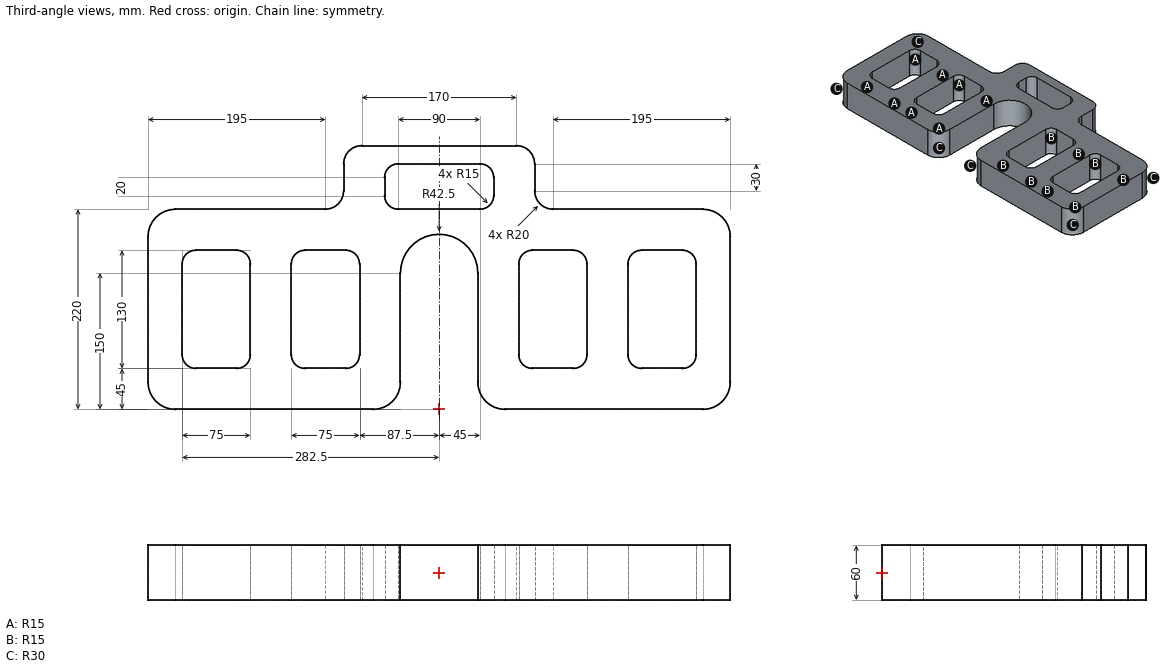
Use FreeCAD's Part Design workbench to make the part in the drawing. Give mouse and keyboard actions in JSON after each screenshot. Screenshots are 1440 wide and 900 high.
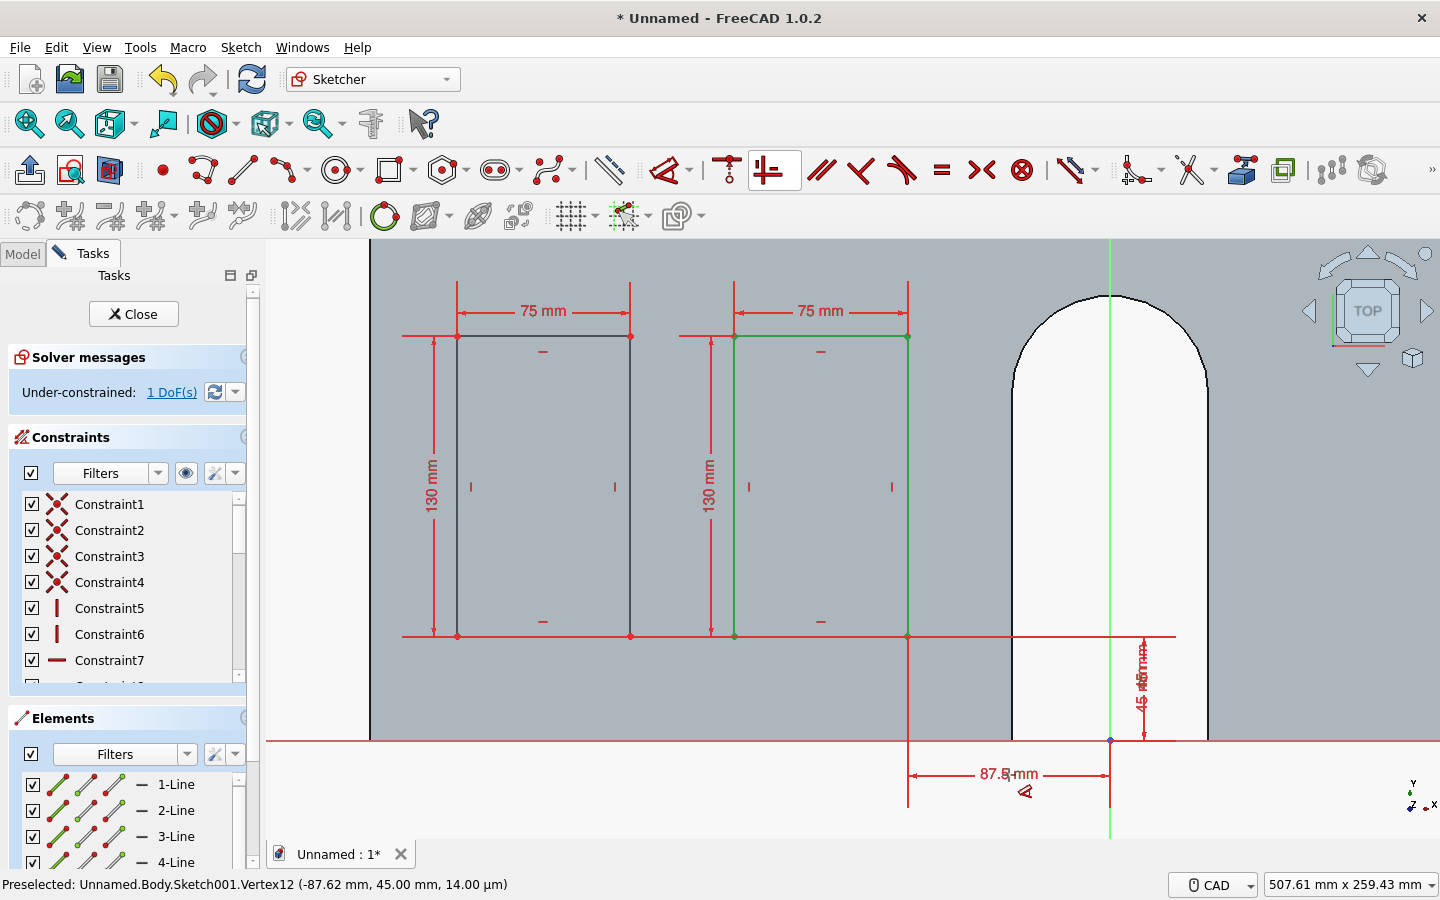
{"action": "left_click", "coordinate": [457, 336]}
{"action": "left_click", "coordinate": [784, 775]}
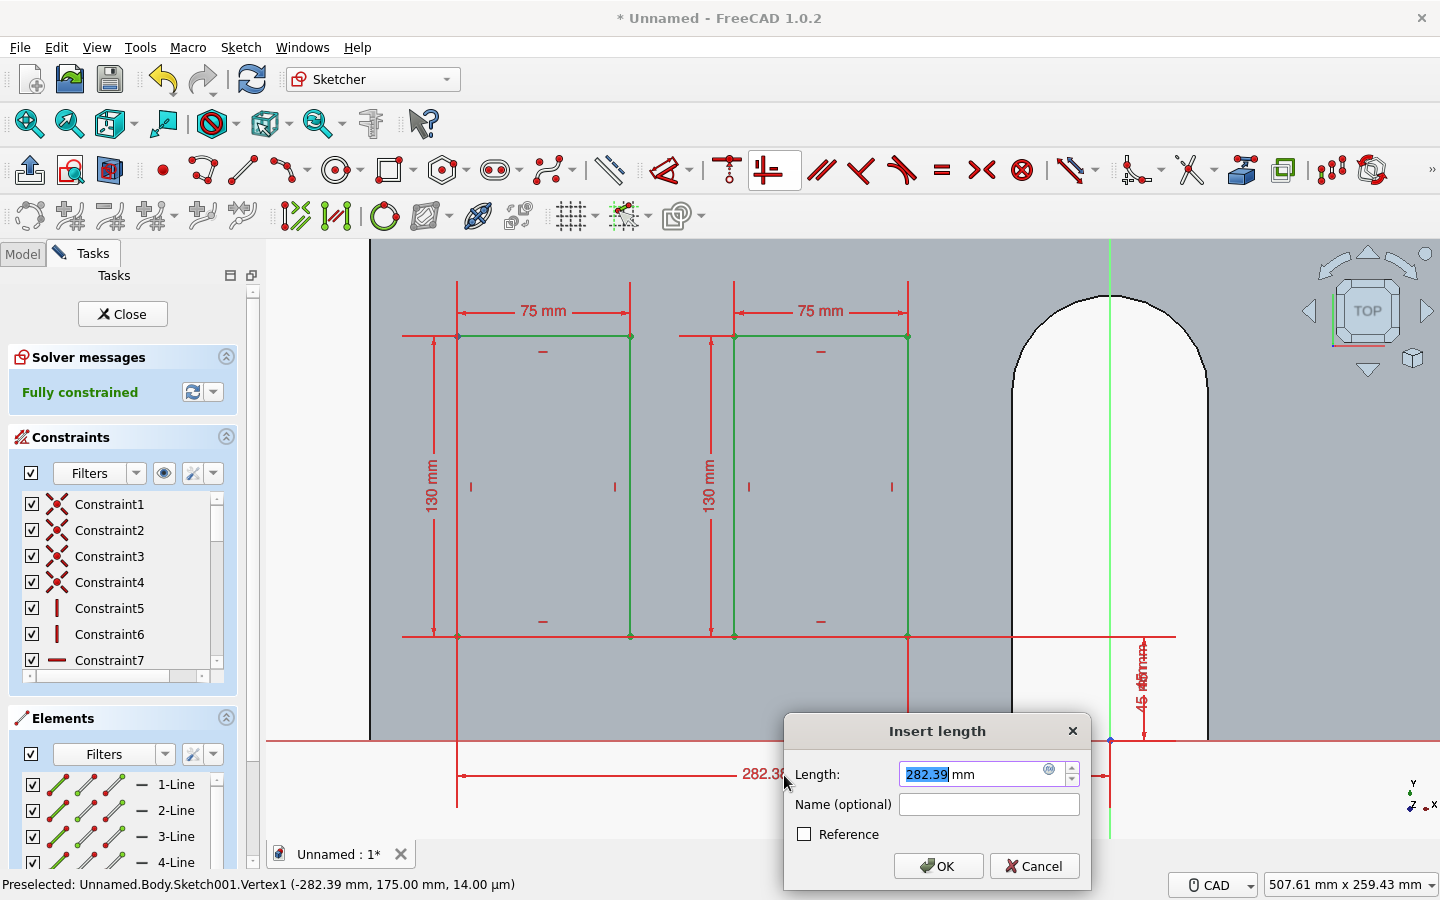
{"action": "type", "text": "282.5"}
{"action": "key", "text": "Return"}
{"action": "key", "text": "Escape"}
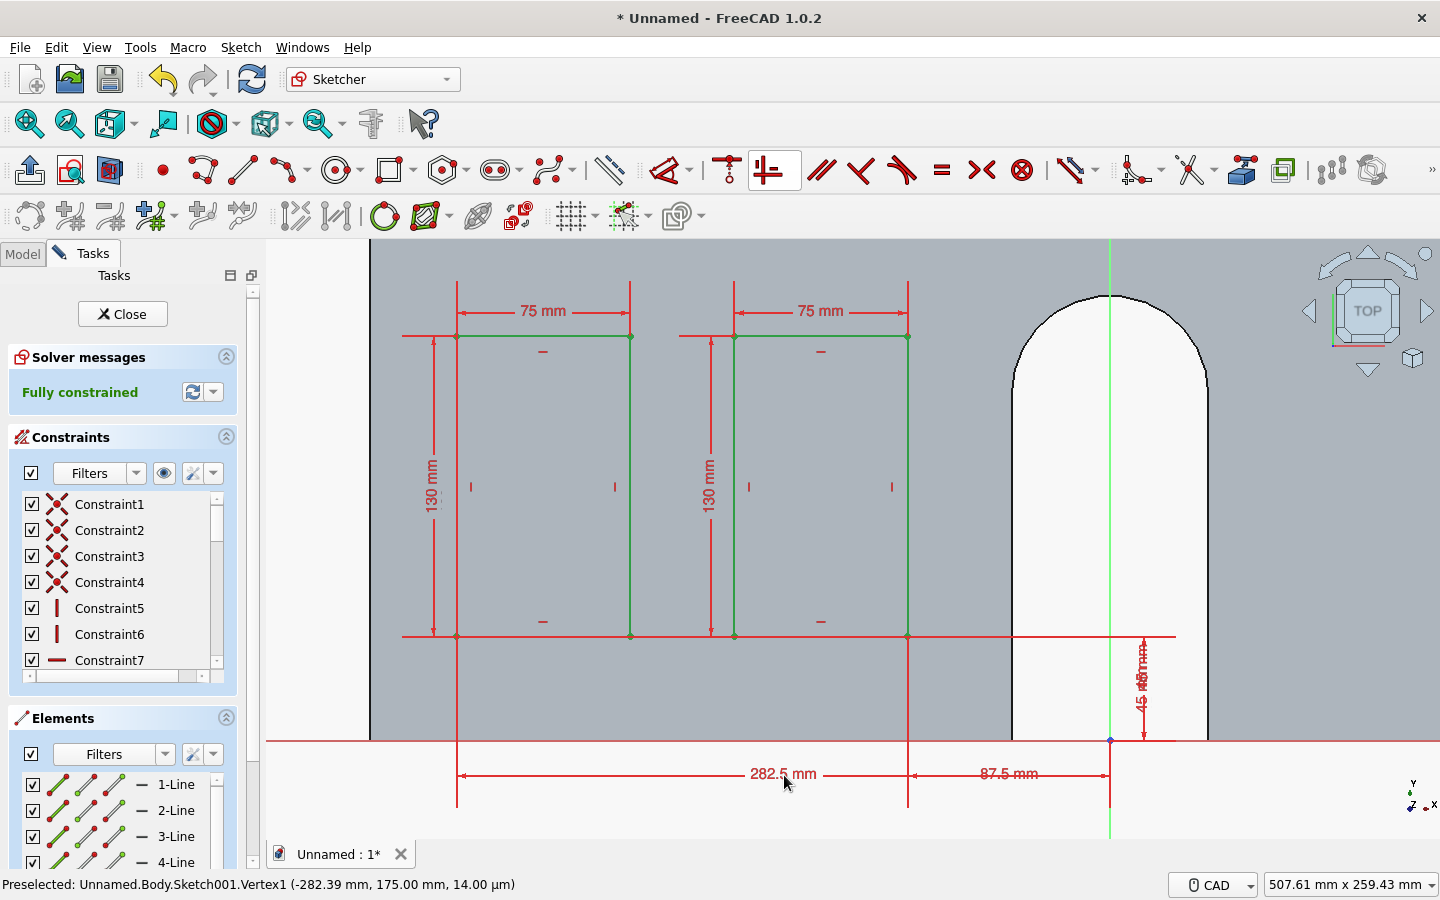
{"action": "left_click", "coordinate": [123, 314]}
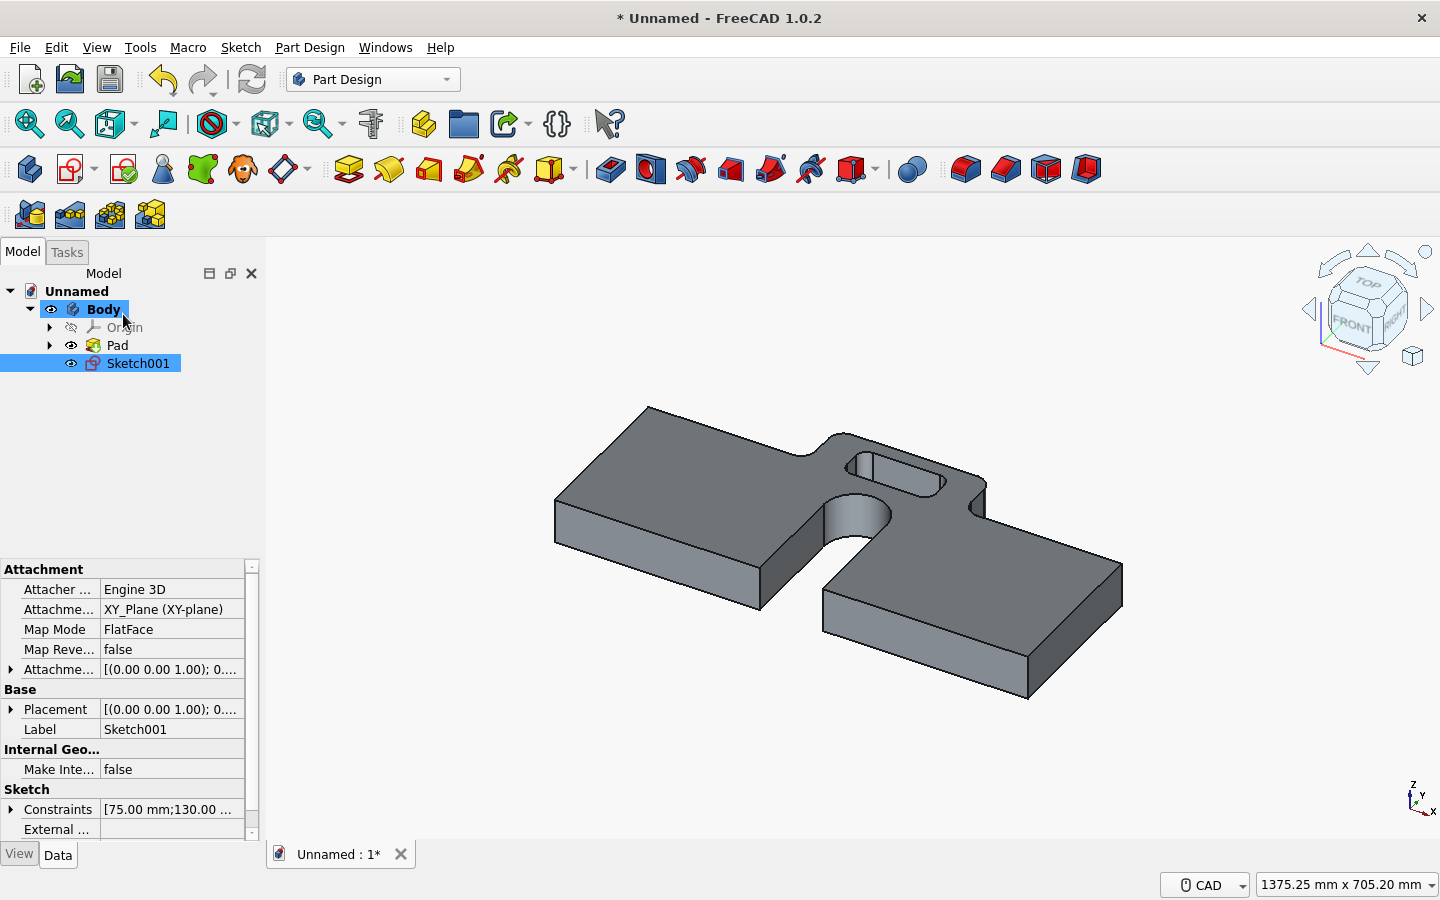
{"action": "left_click", "coordinate": [612, 170]}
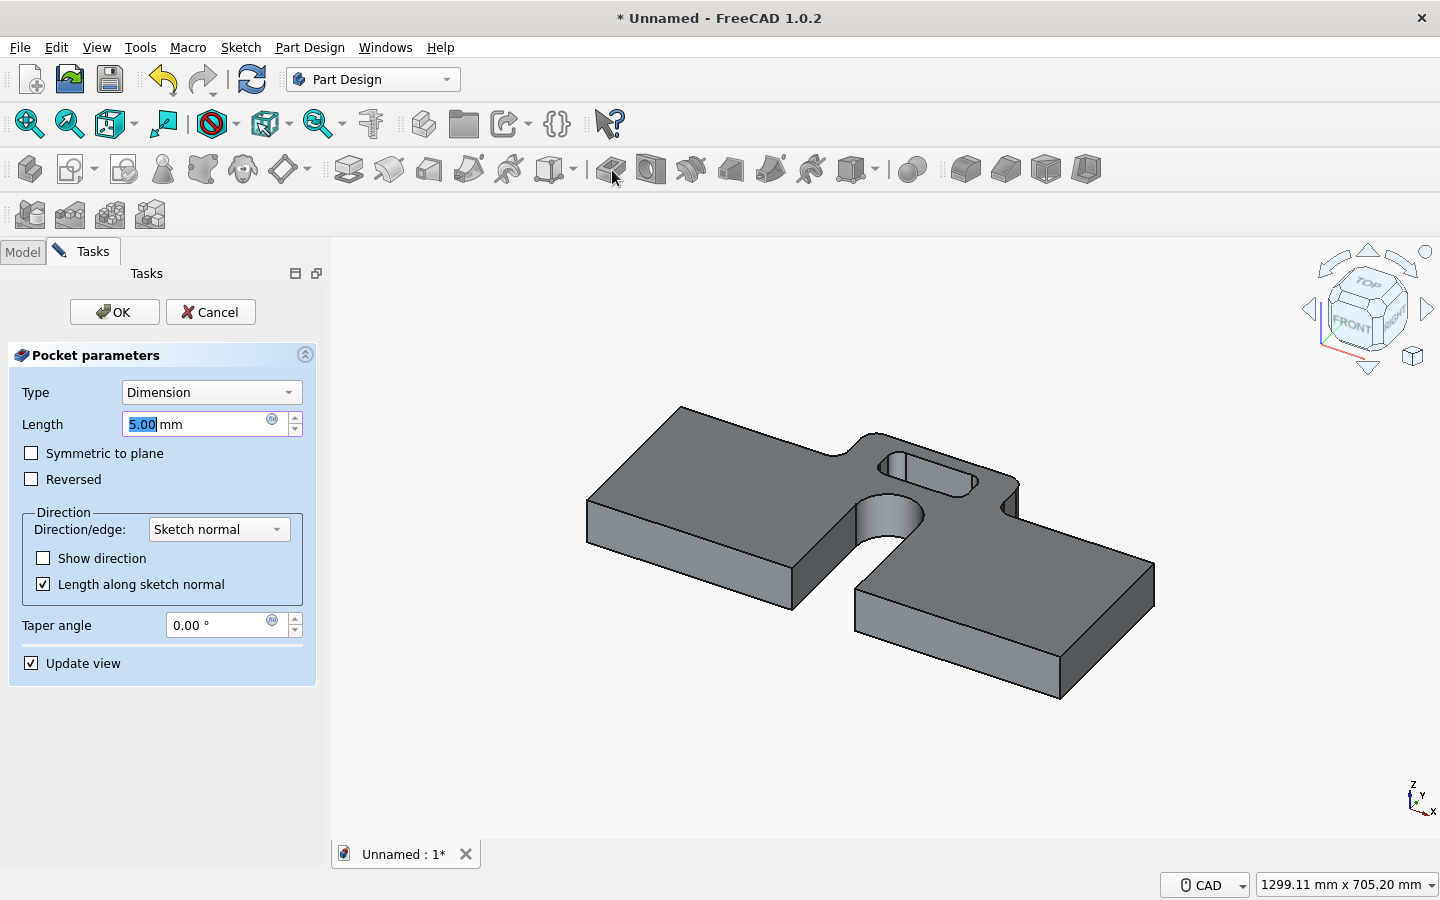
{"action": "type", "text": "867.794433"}
{"action": "key", "text": "Tab"}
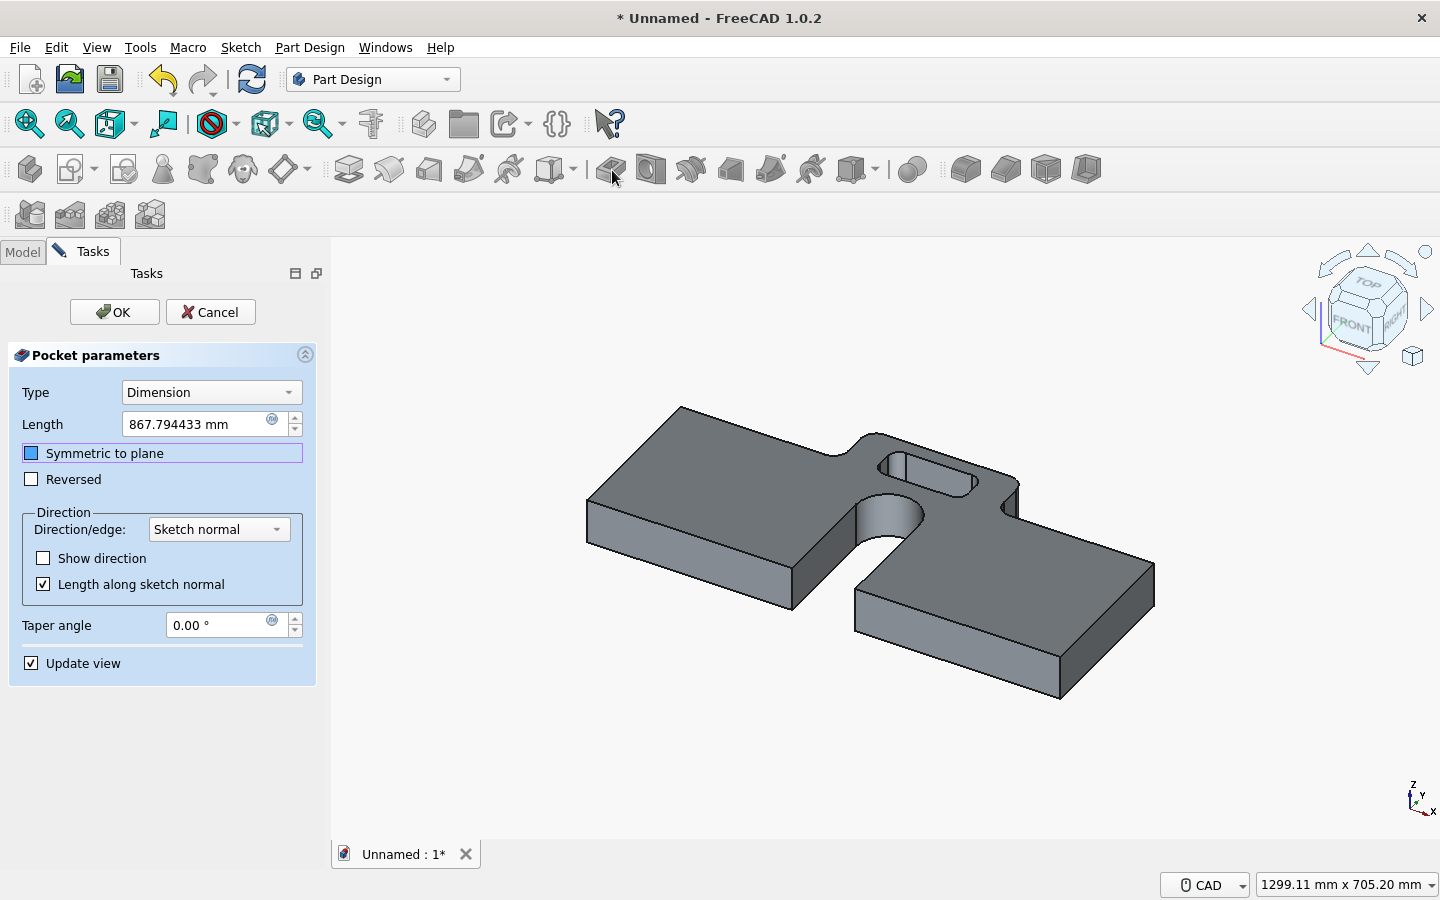
{"action": "left_click", "coordinate": [30, 453]}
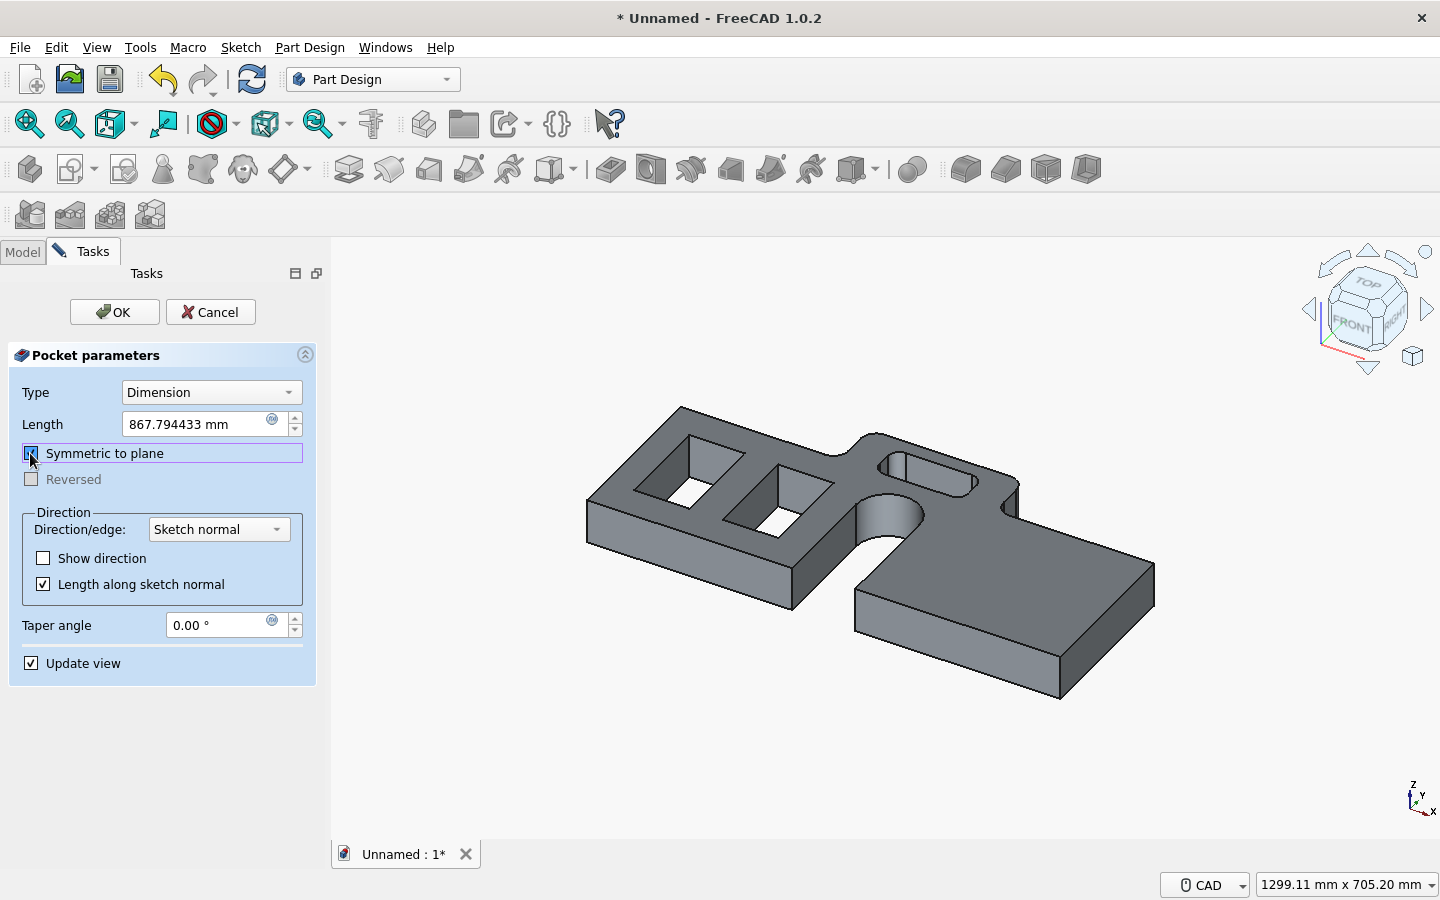
{"action": "left_click", "coordinate": [115, 312]}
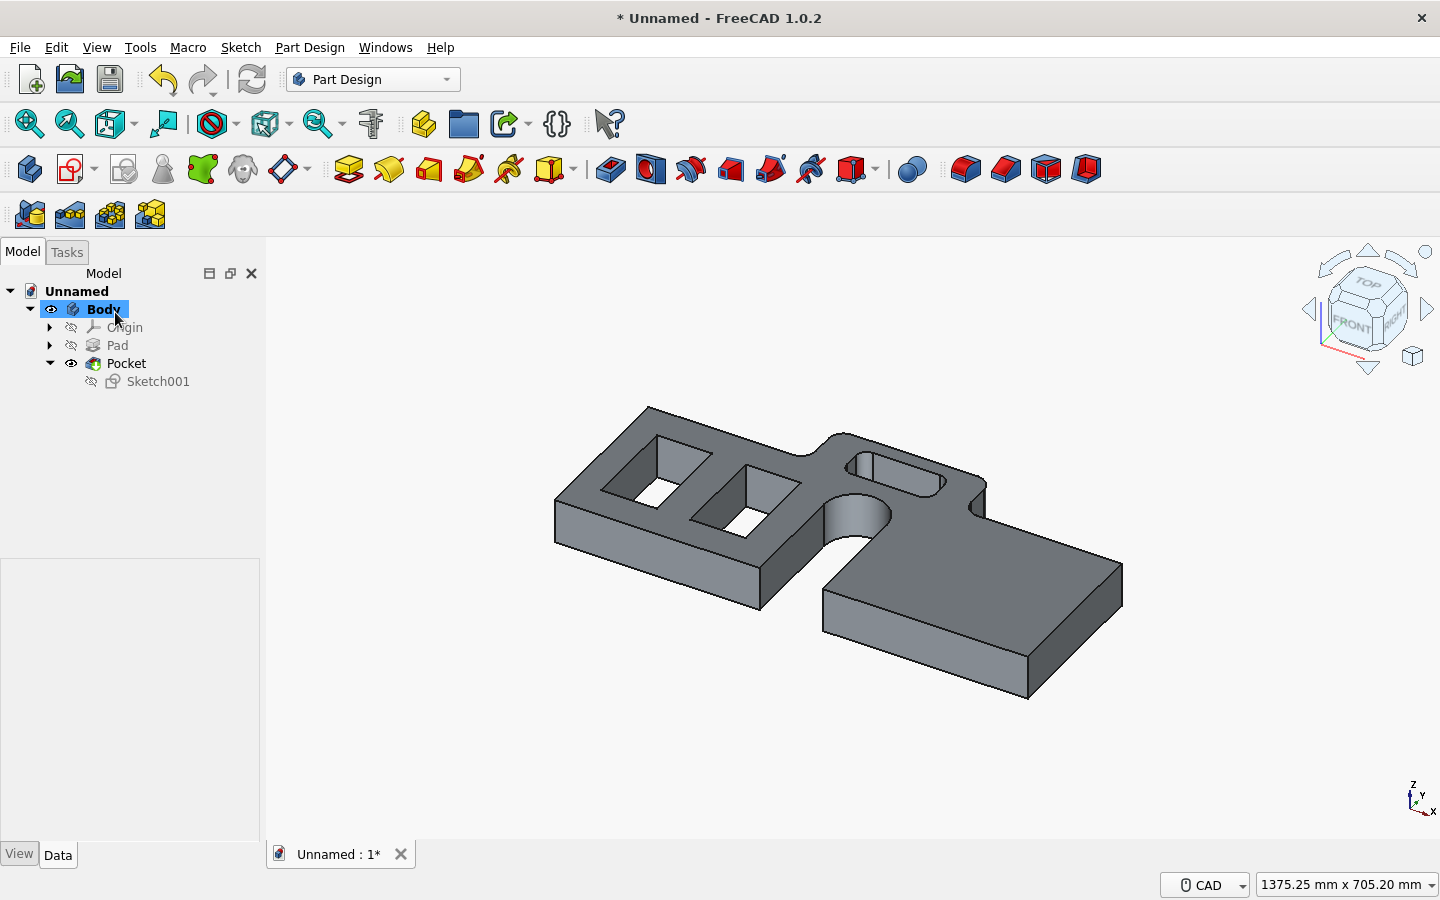
{"action": "key", "text": "0"}